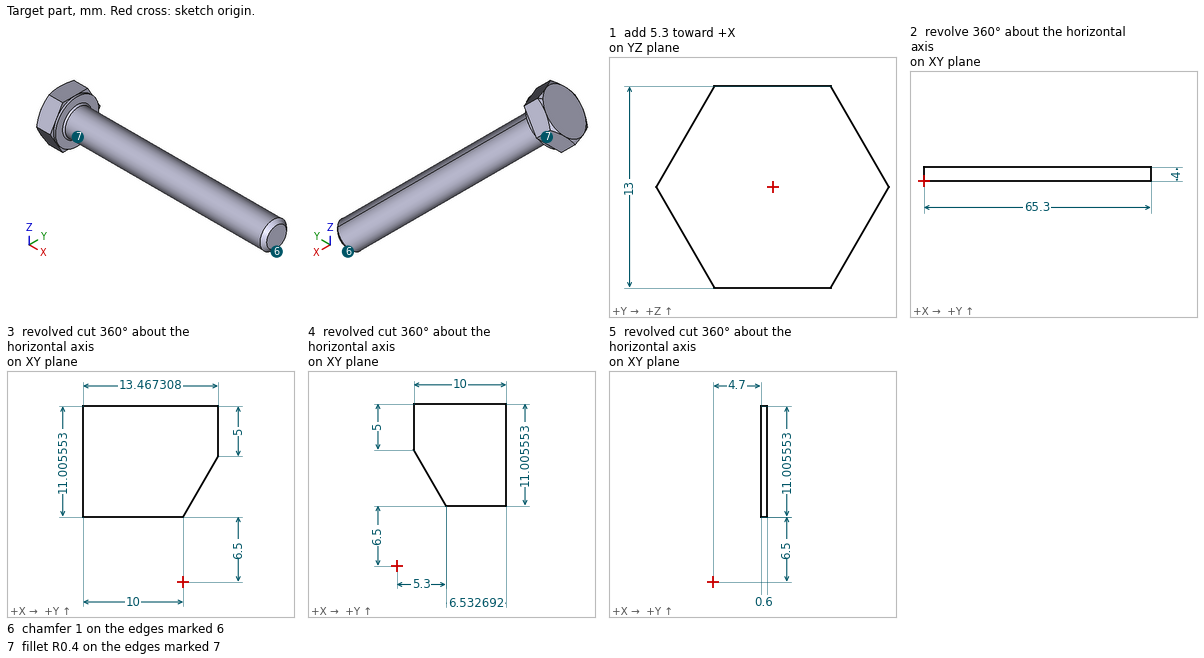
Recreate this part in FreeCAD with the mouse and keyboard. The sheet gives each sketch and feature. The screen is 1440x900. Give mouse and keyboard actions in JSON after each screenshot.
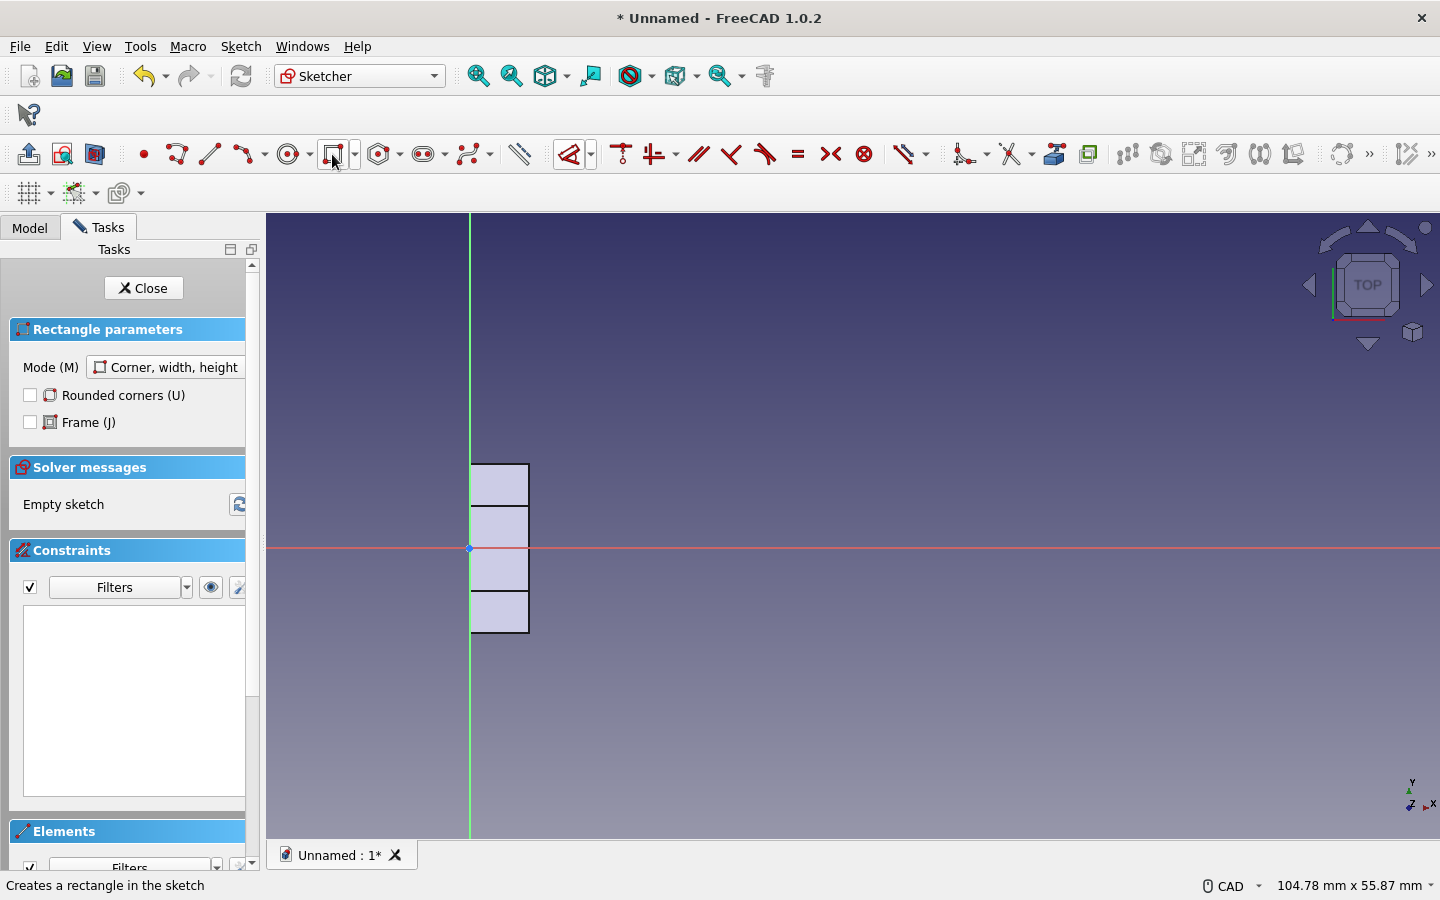
{"action": "left_click", "coordinate": [470, 548]}
{"action": "left_click", "coordinate": [1202, 504]}
{"action": "key", "text": "Escape"}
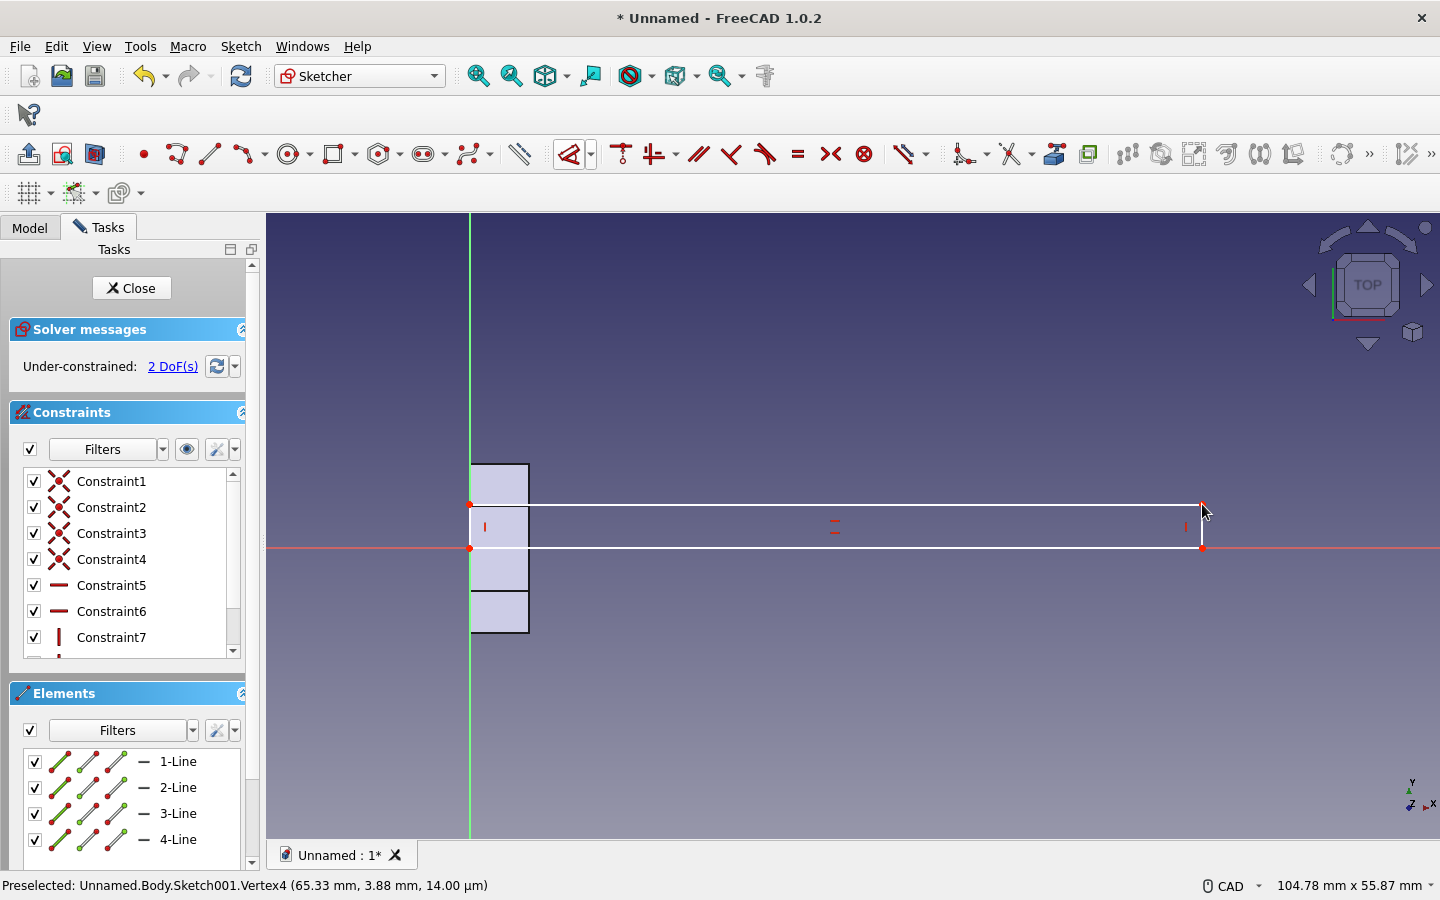
{"action": "left_click", "coordinate": [1202, 535]}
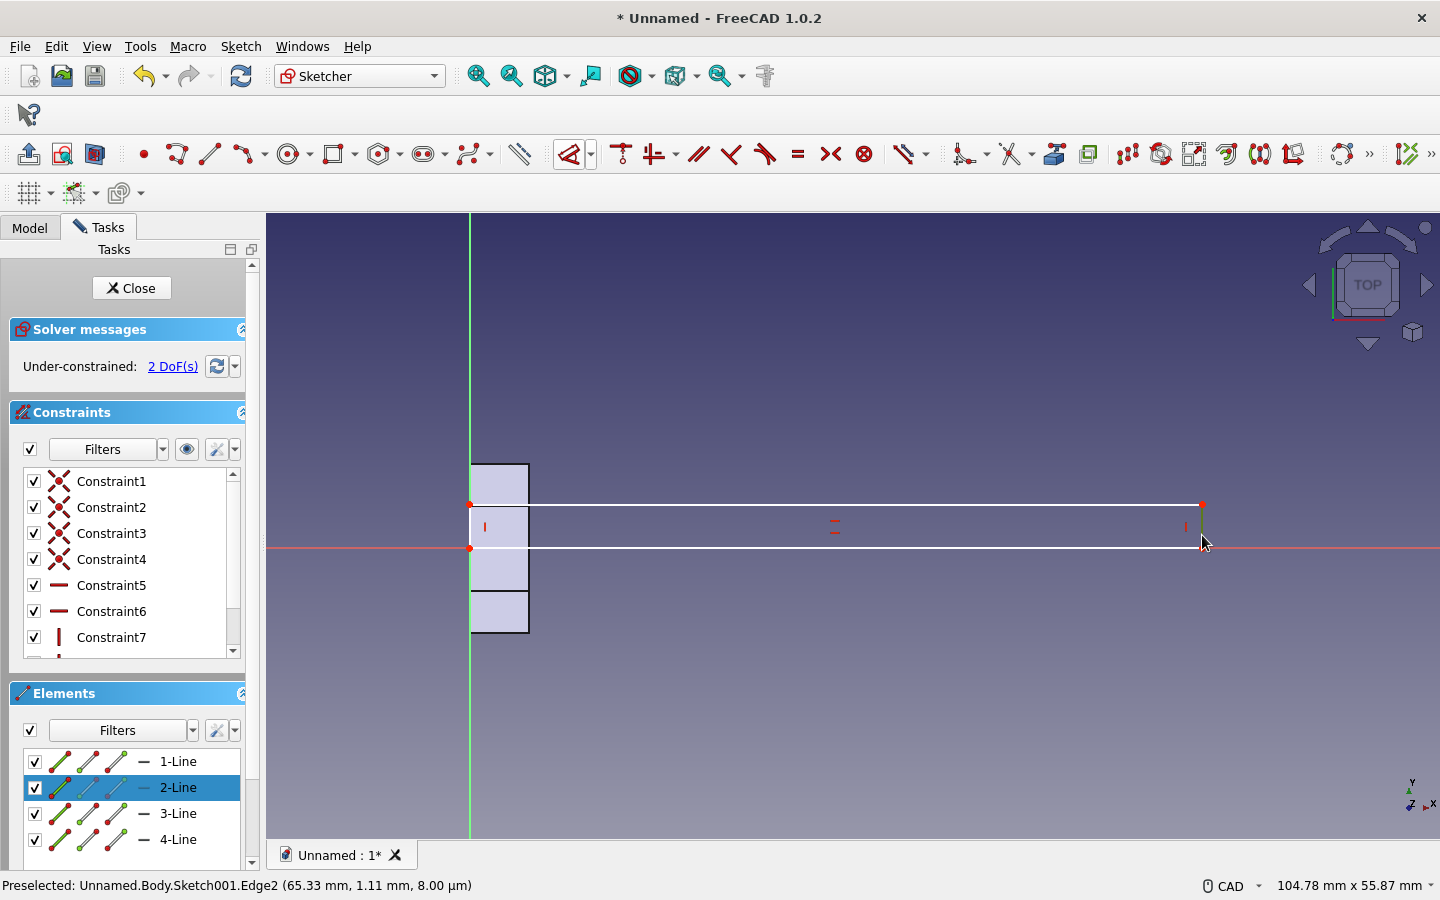
{"action": "left_click", "coordinate": [590, 154]}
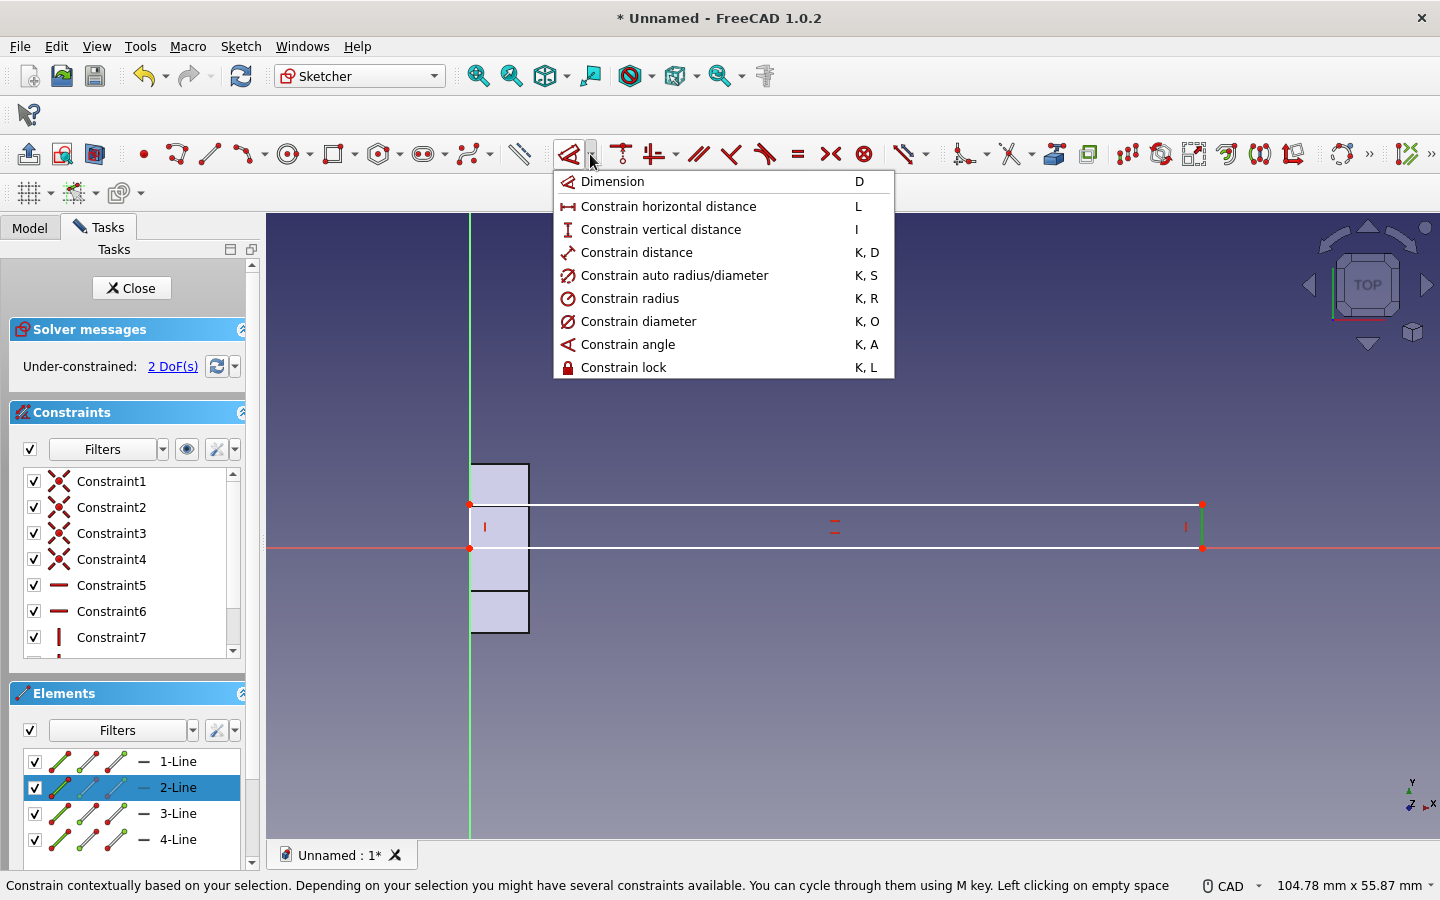
{"action": "left_click", "coordinate": [724, 230]}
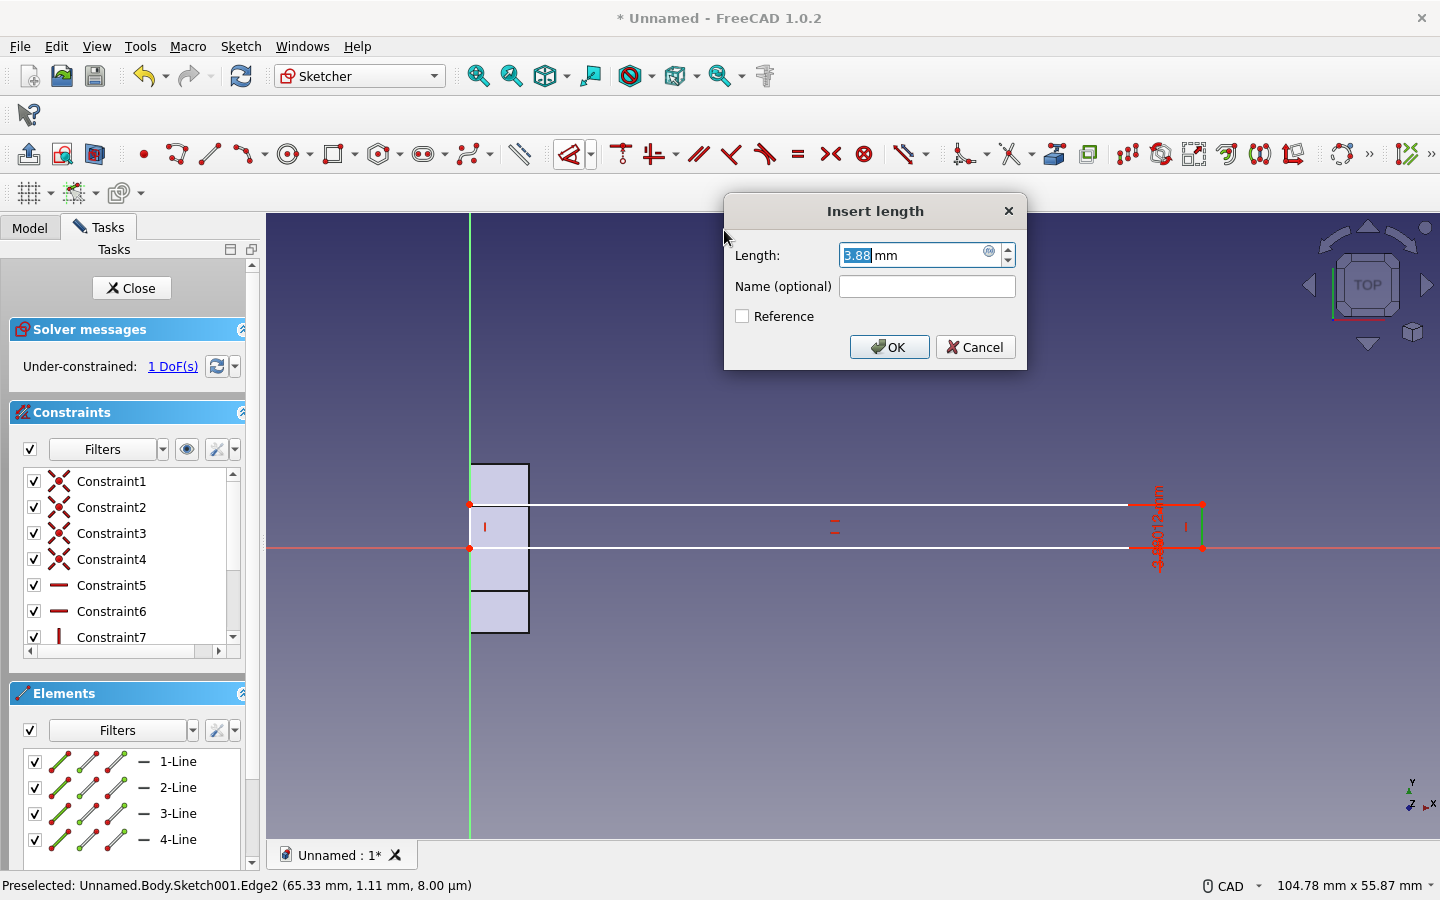
{"action": "type", "text": "4"}
{"action": "key", "text": "Return"}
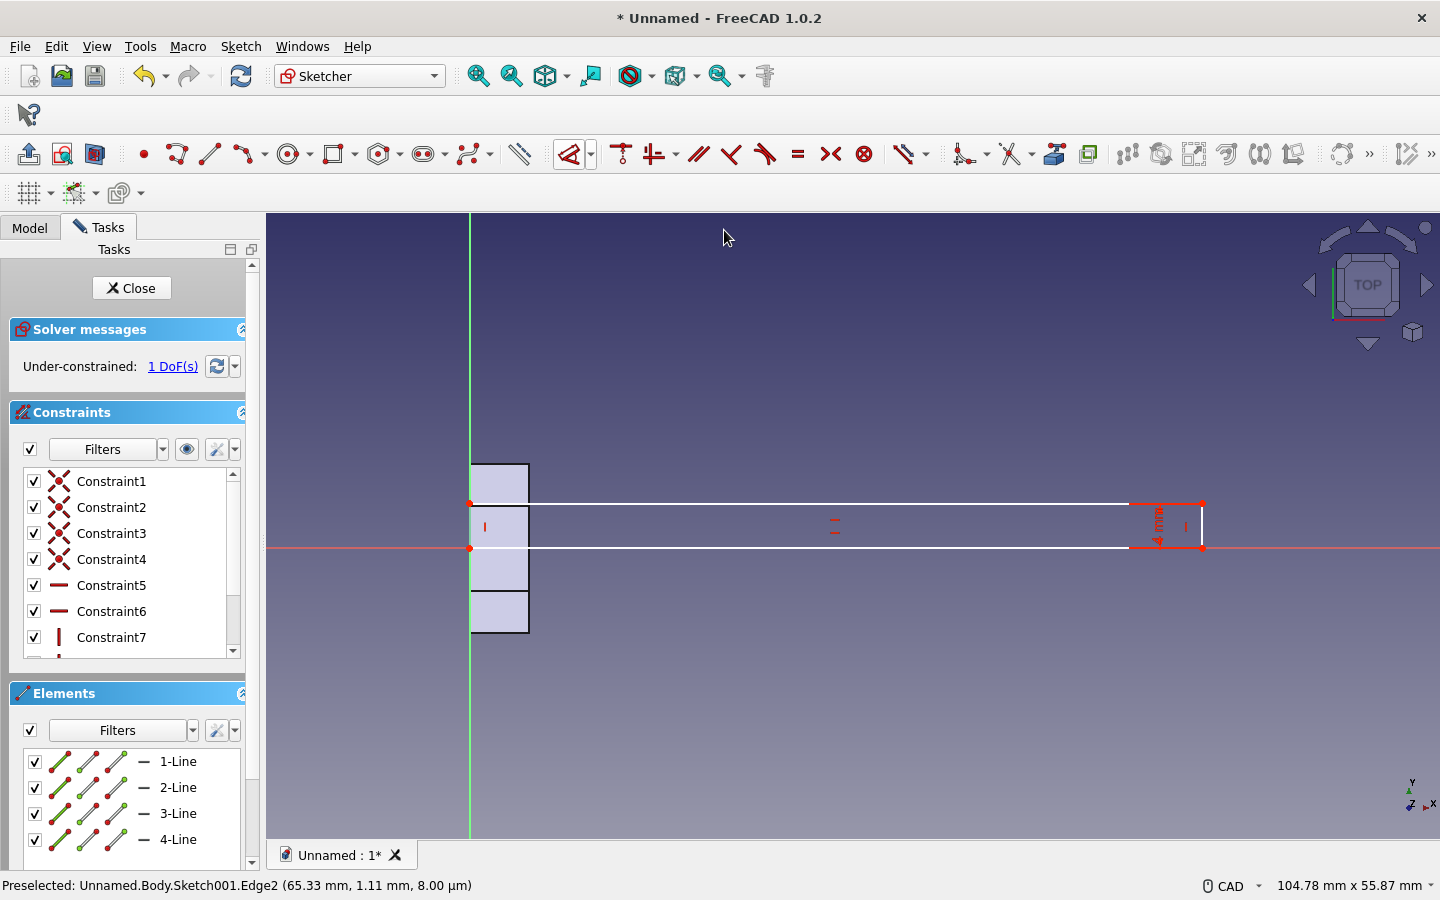
{"action": "left_click", "coordinate": [690, 548]}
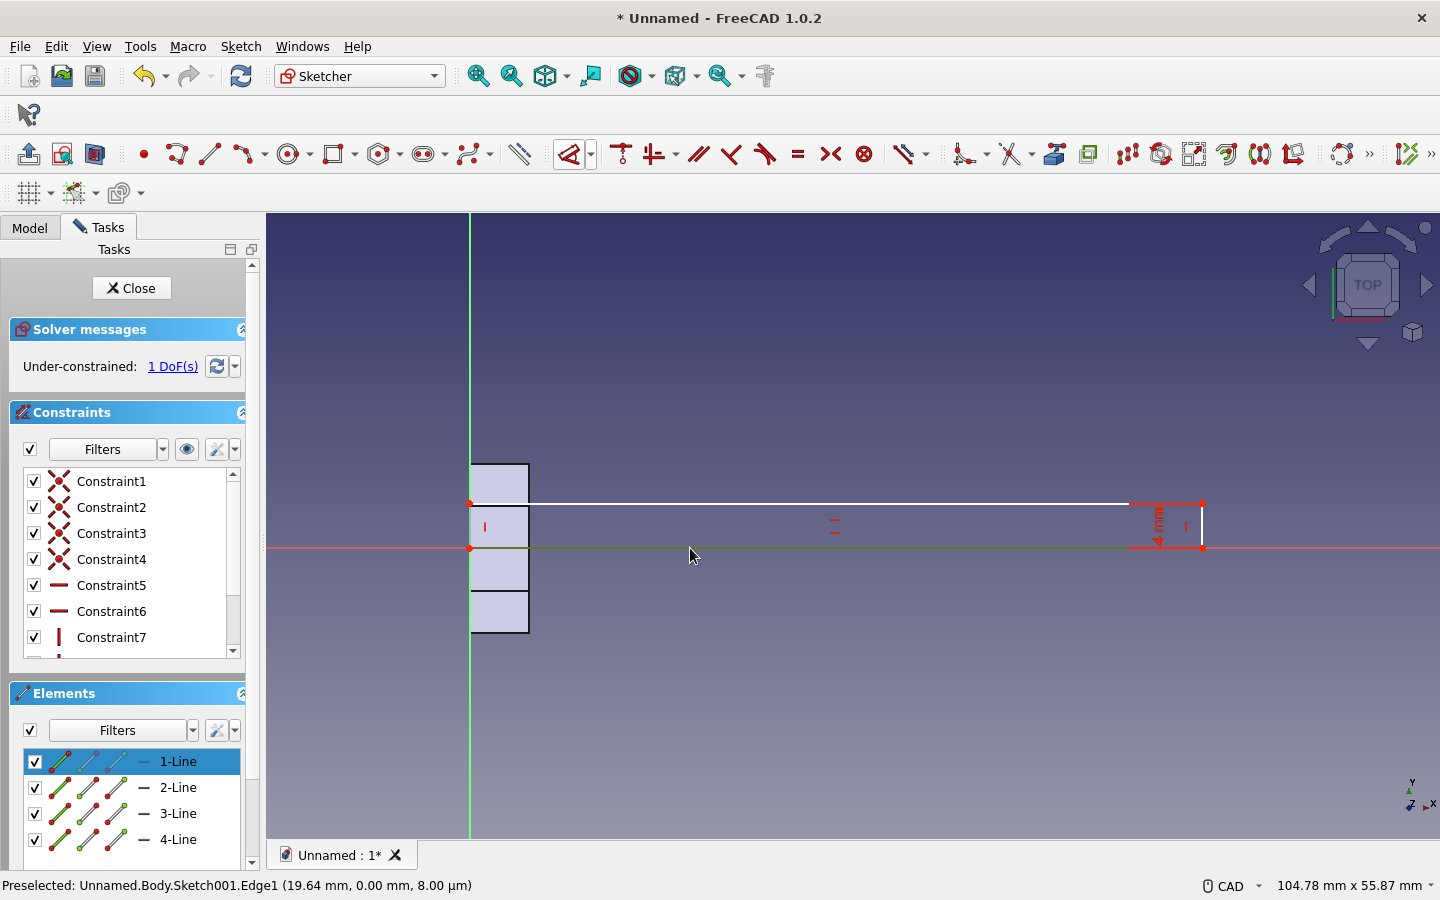
{"action": "left_click", "coordinate": [590, 154]}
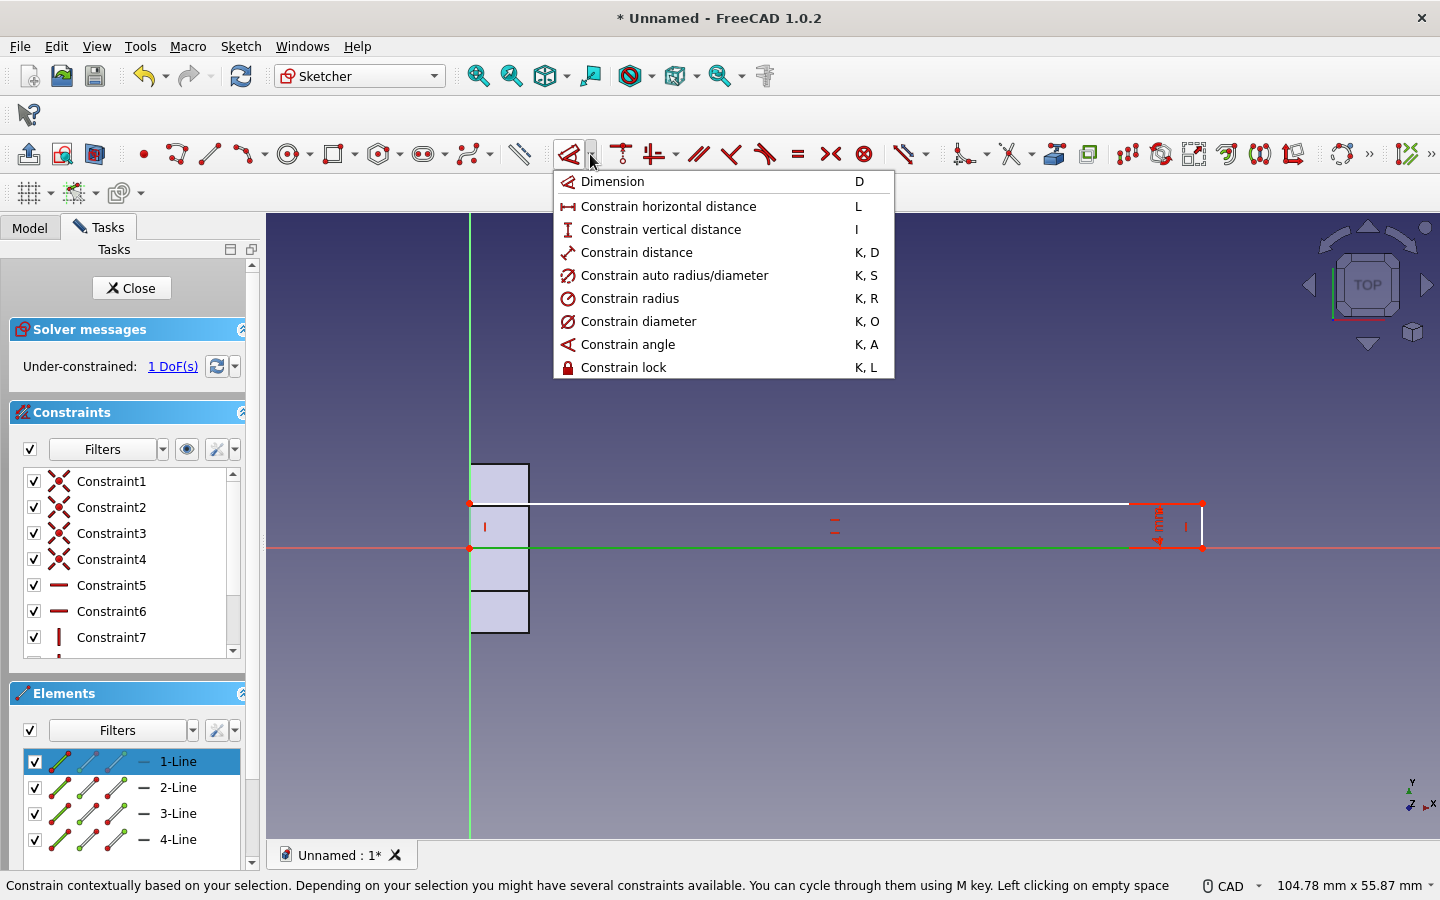
{"action": "left_click", "coordinate": [724, 206]}